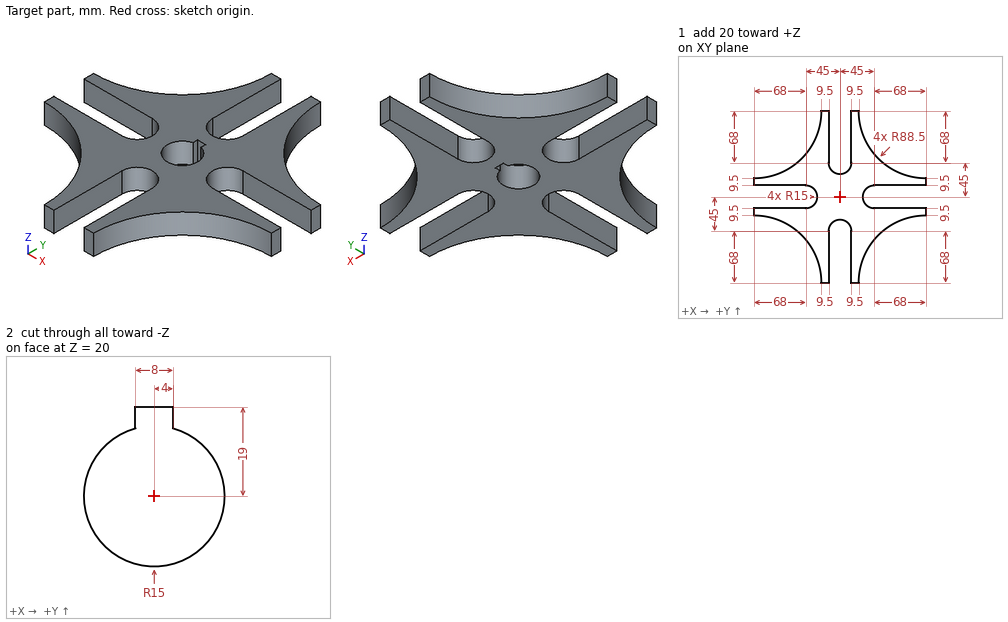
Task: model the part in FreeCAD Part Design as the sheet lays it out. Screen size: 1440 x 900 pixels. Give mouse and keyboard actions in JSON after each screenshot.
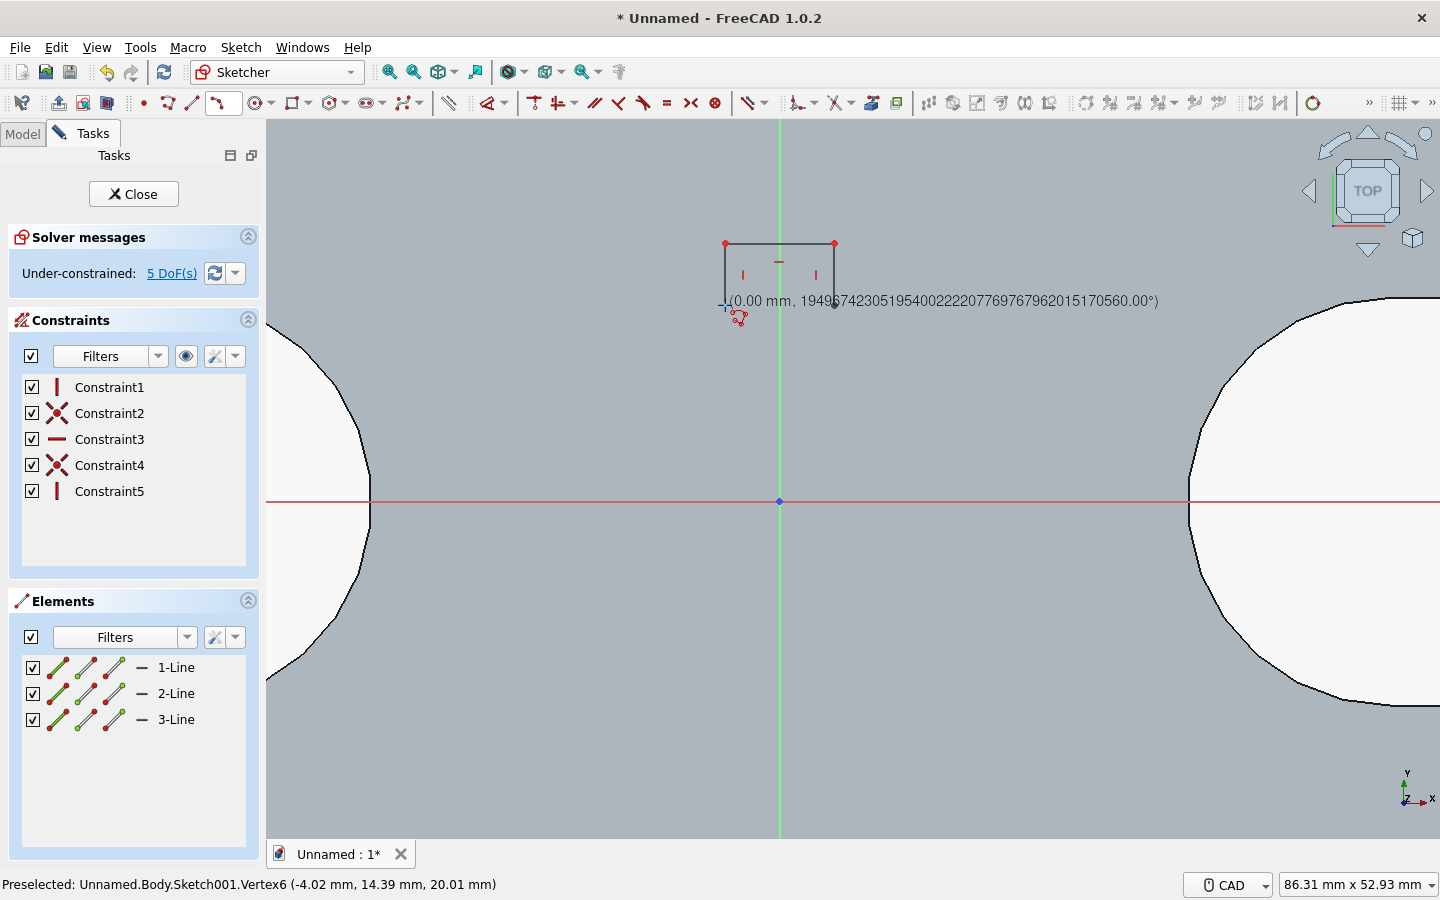
{"action": "left_click", "coordinate": [218, 104]}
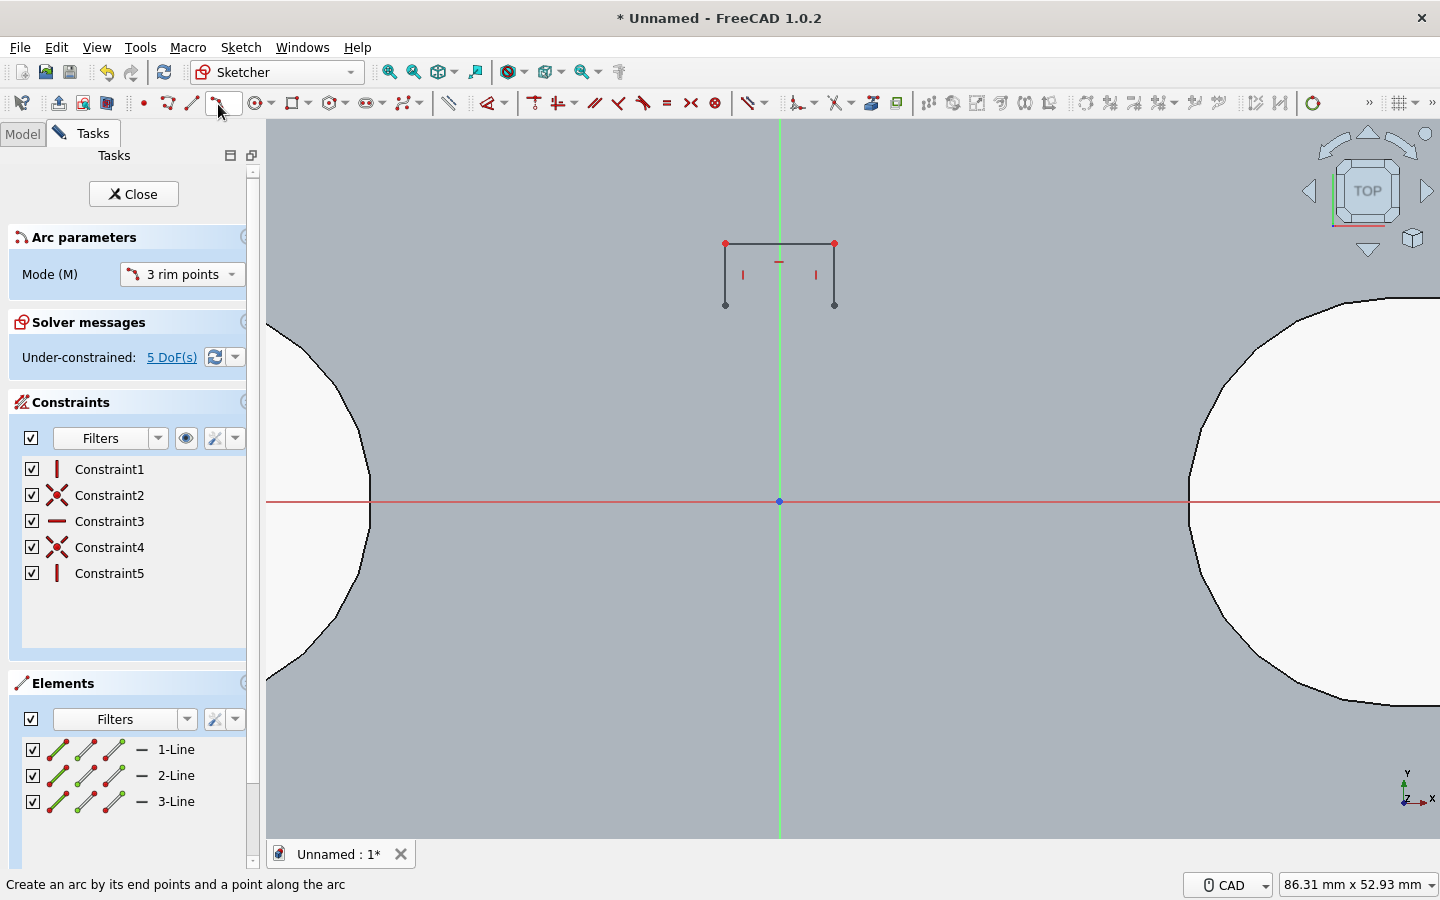
{"action": "left_click", "coordinate": [725, 306]}
{"action": "left_click", "coordinate": [834, 306]}
{"action": "left_click", "coordinate": [669, 673]}
{"action": "key", "text": "Escape"}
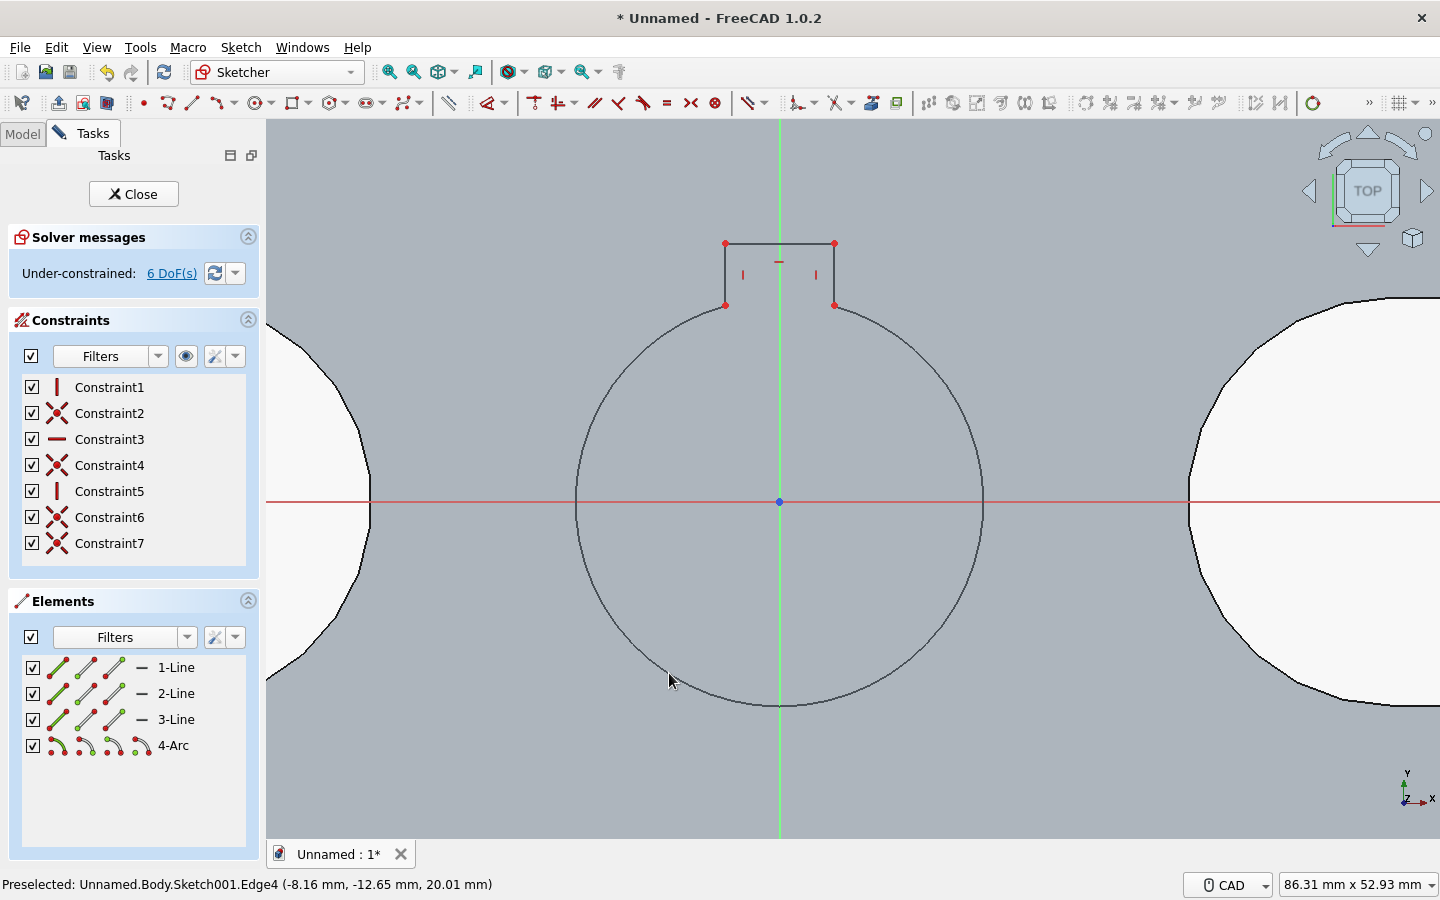
{"action": "left_click_drag", "start_coordinate": [770, 492], "coordinate": [790, 513]}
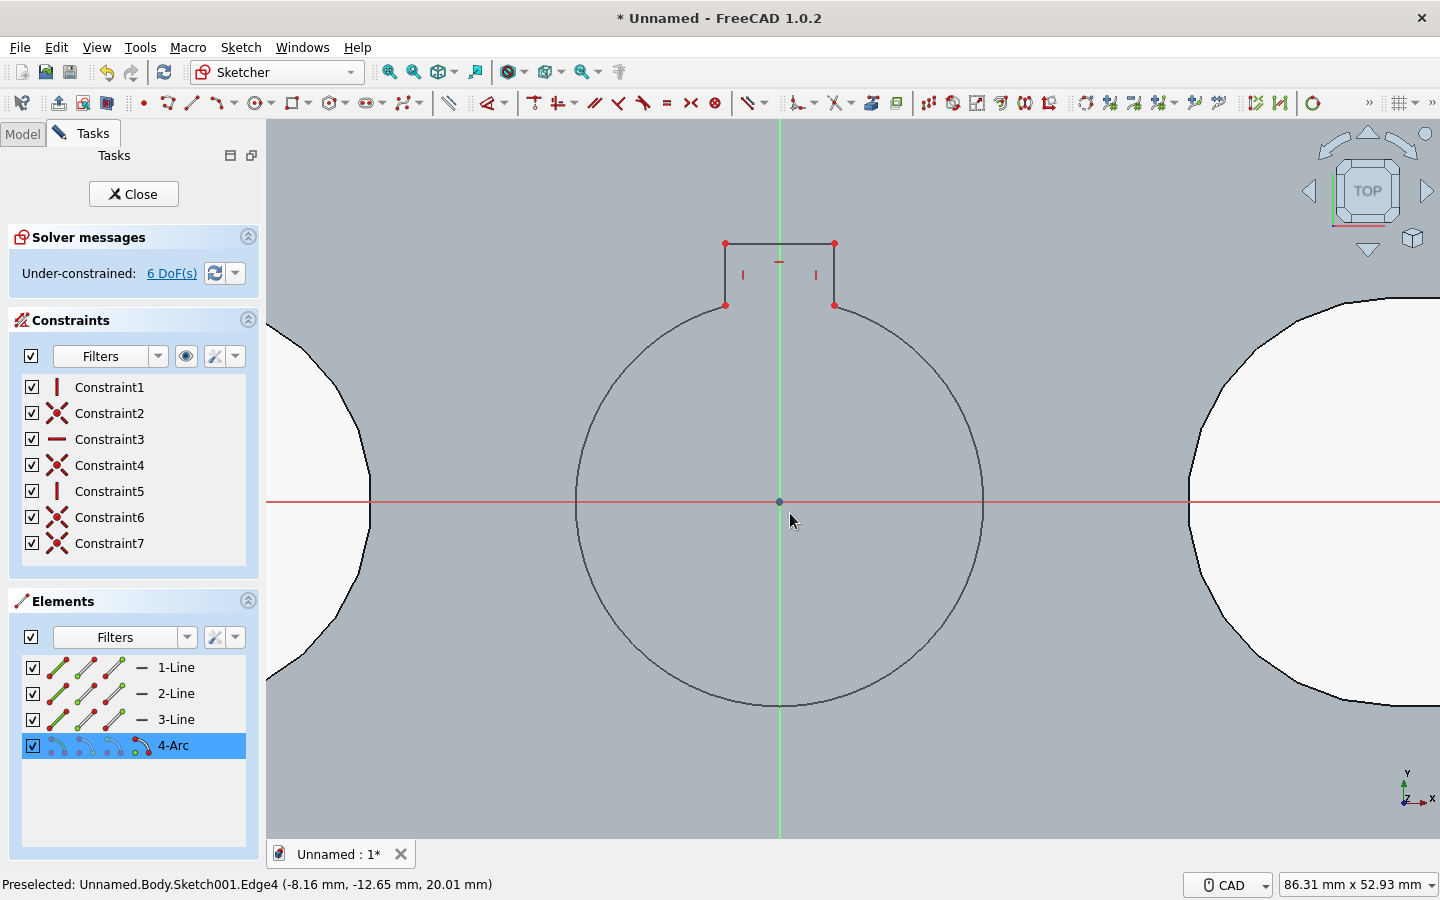
{"action": "left_click", "coordinate": [534, 104]}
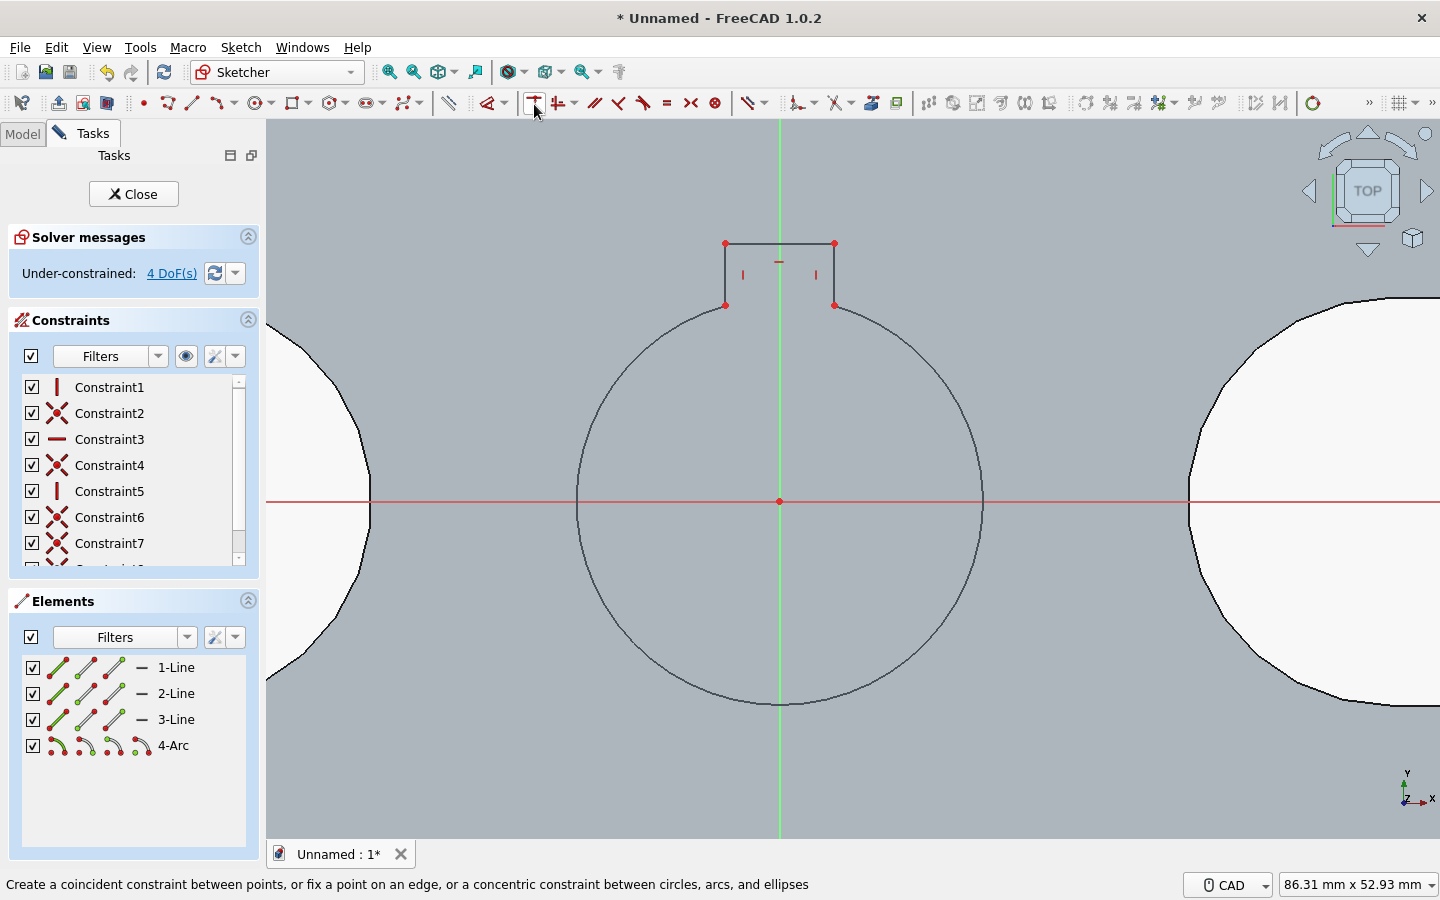
{"action": "left_click", "coordinate": [488, 104]}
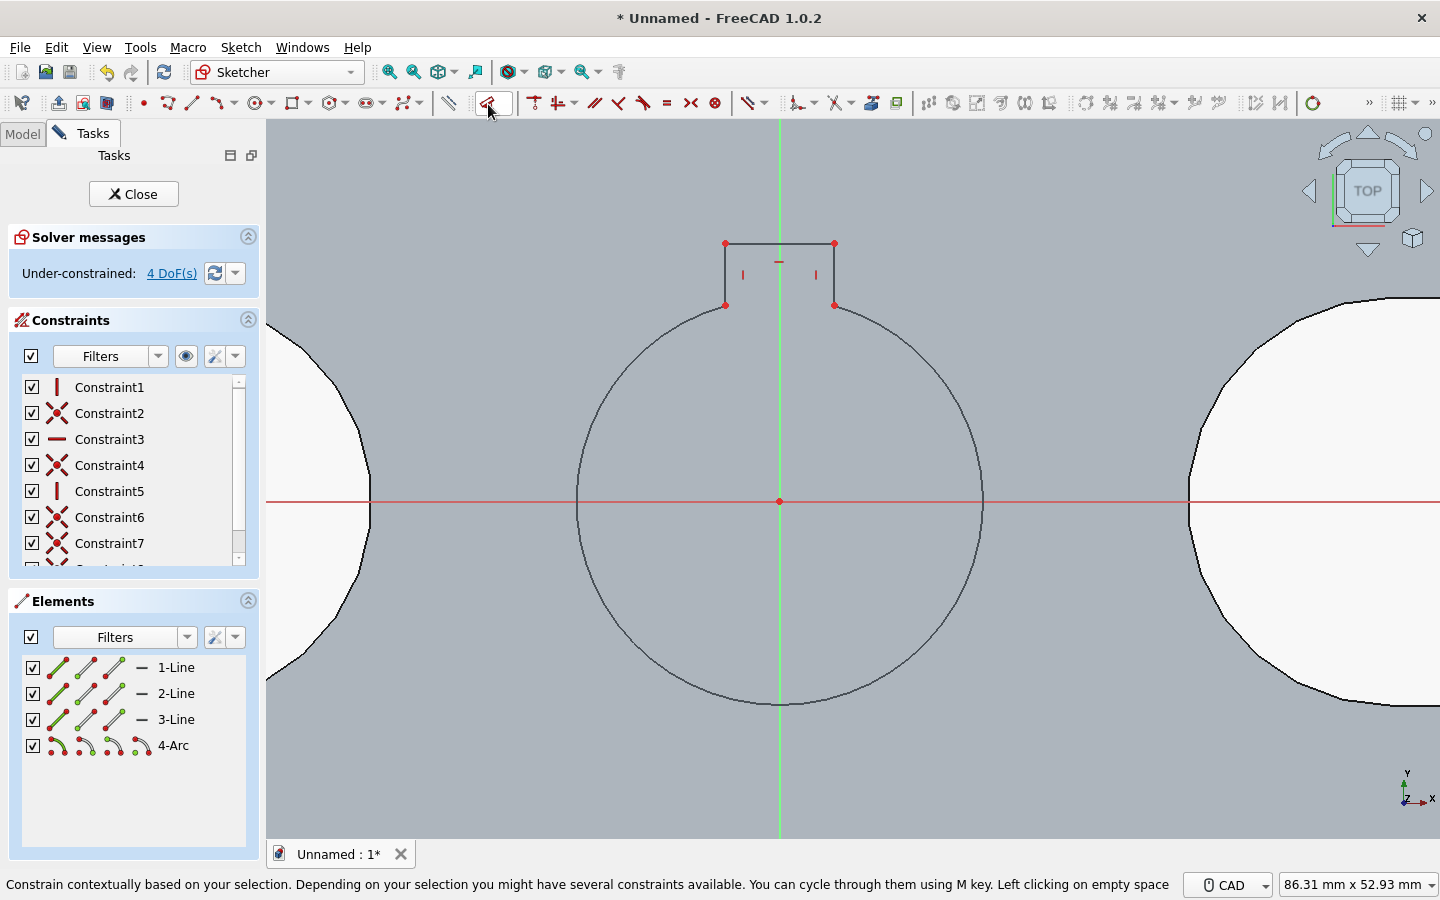
{"action": "left_click", "coordinate": [594, 585]}
{"action": "left_click", "coordinate": [565, 598]}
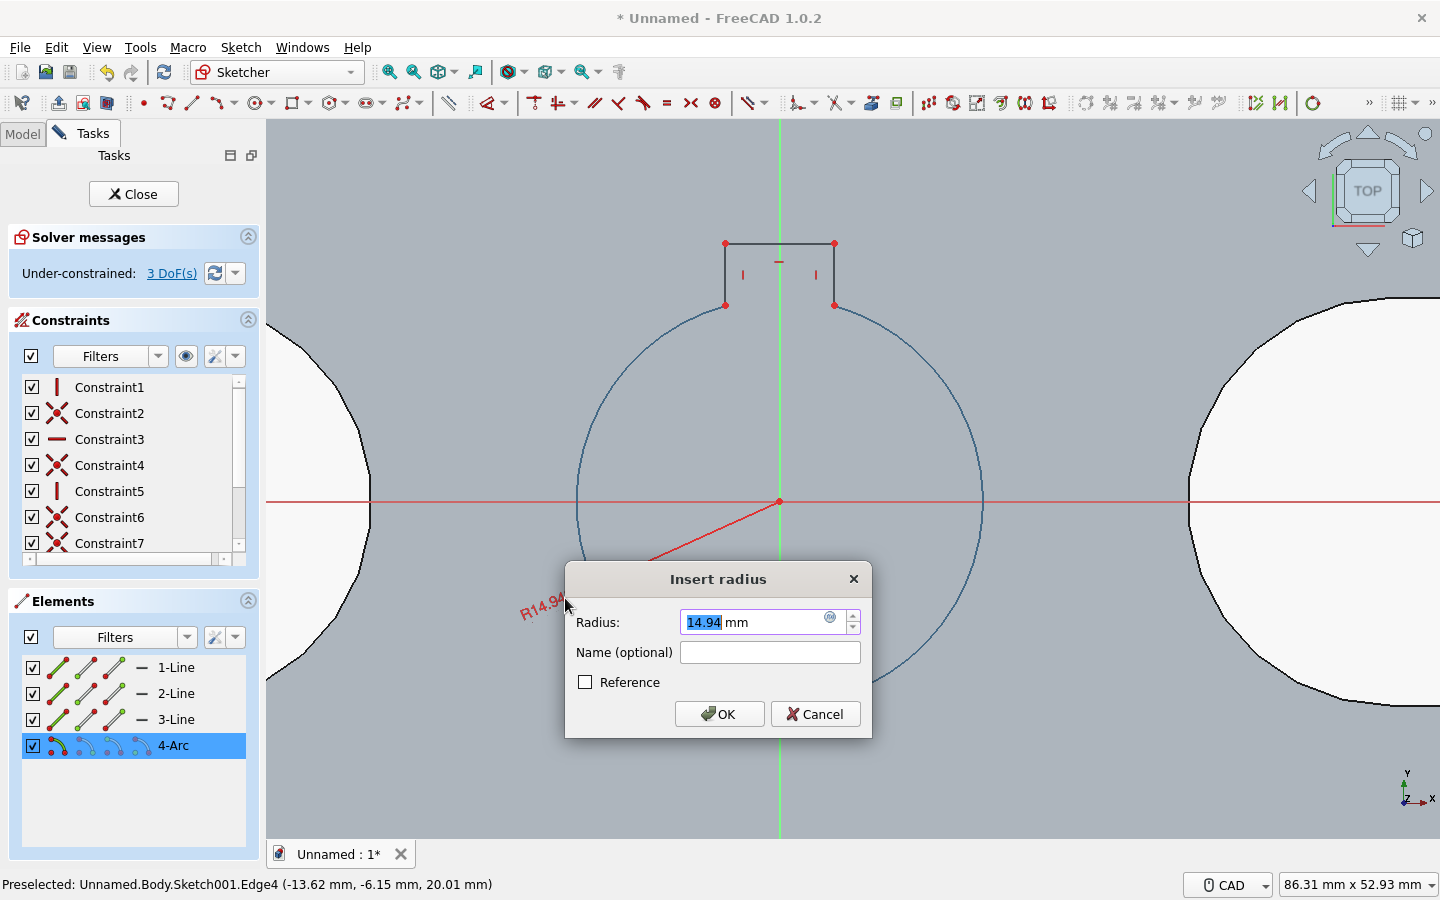
{"action": "type", "text": "15"}
{"action": "key", "text": "Return"}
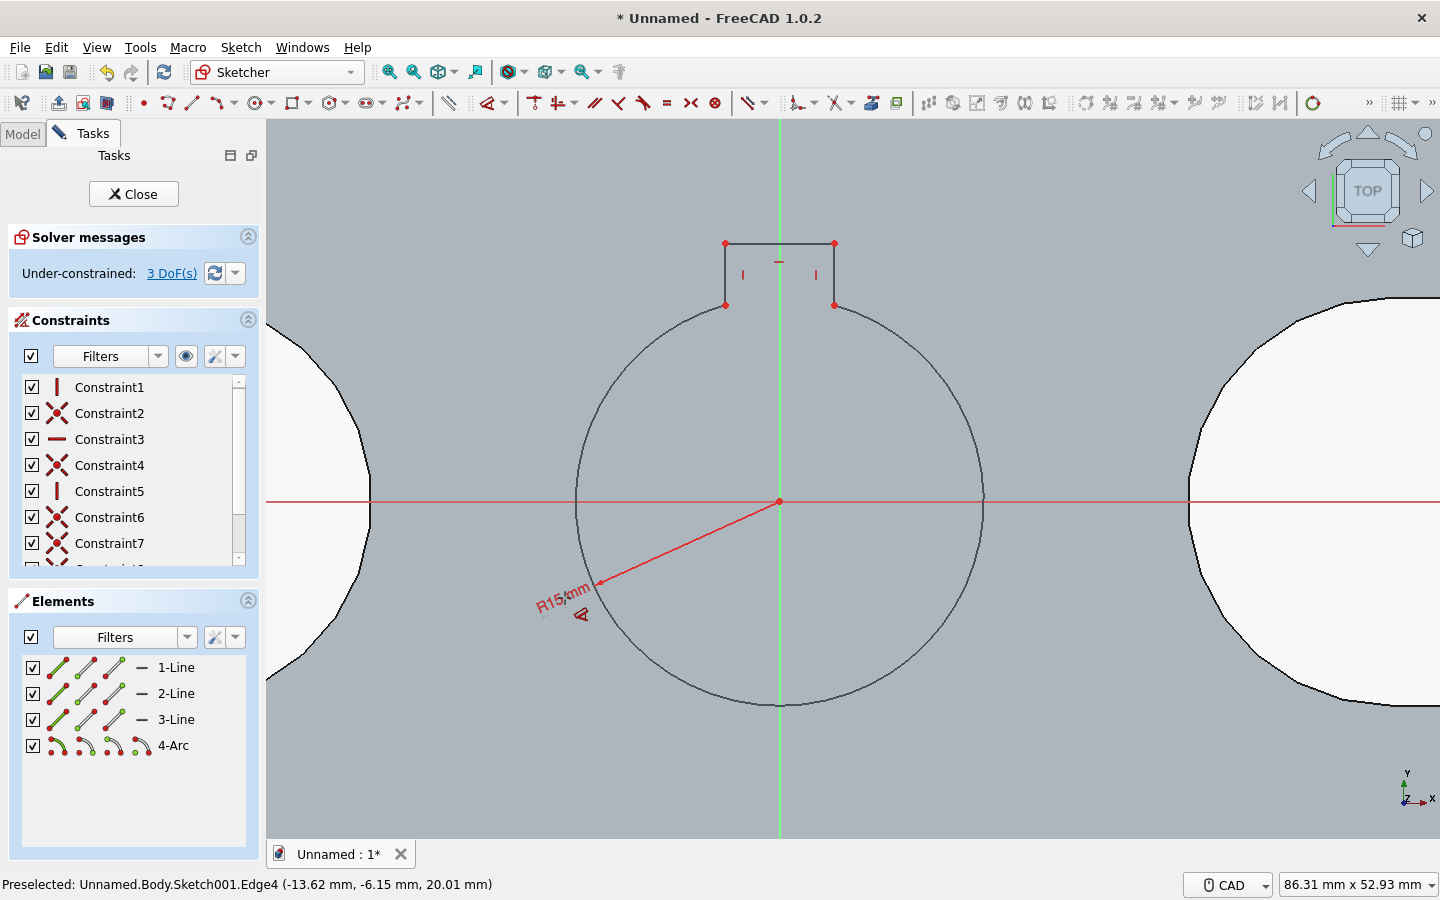
{"action": "left_click", "coordinate": [801, 244]}
{"action": "left_click", "coordinate": [754, 210]}